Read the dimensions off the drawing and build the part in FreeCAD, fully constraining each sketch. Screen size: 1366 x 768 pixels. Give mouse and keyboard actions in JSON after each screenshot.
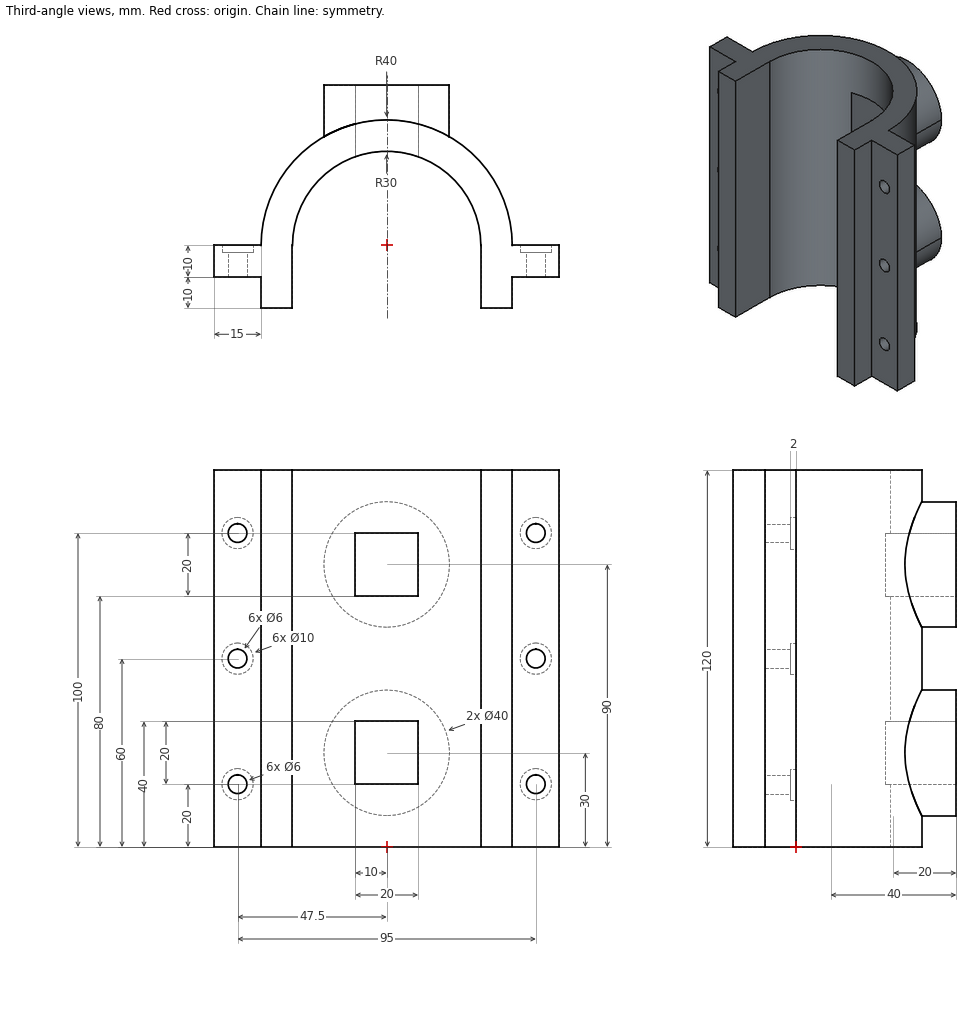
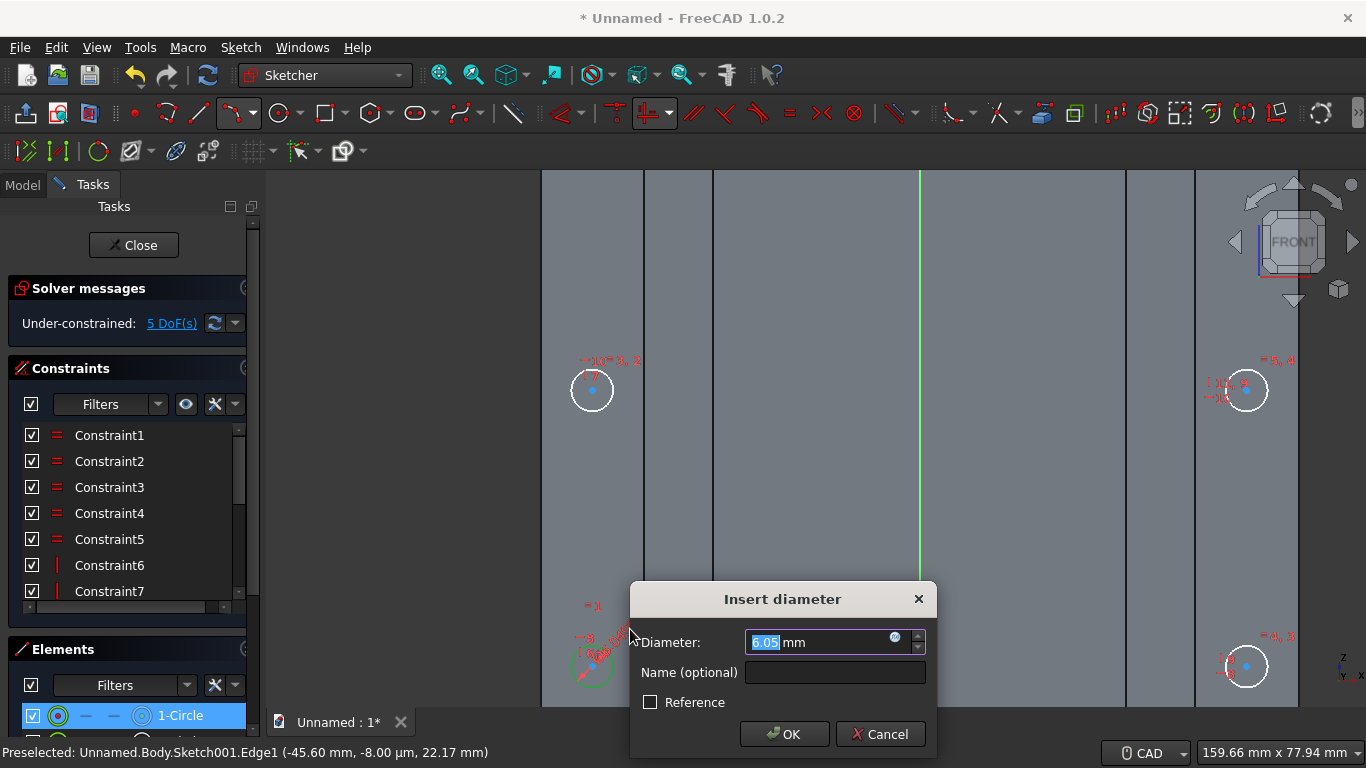
{"action": "type", "text": "6"}
{"action": "key", "text": "Return"}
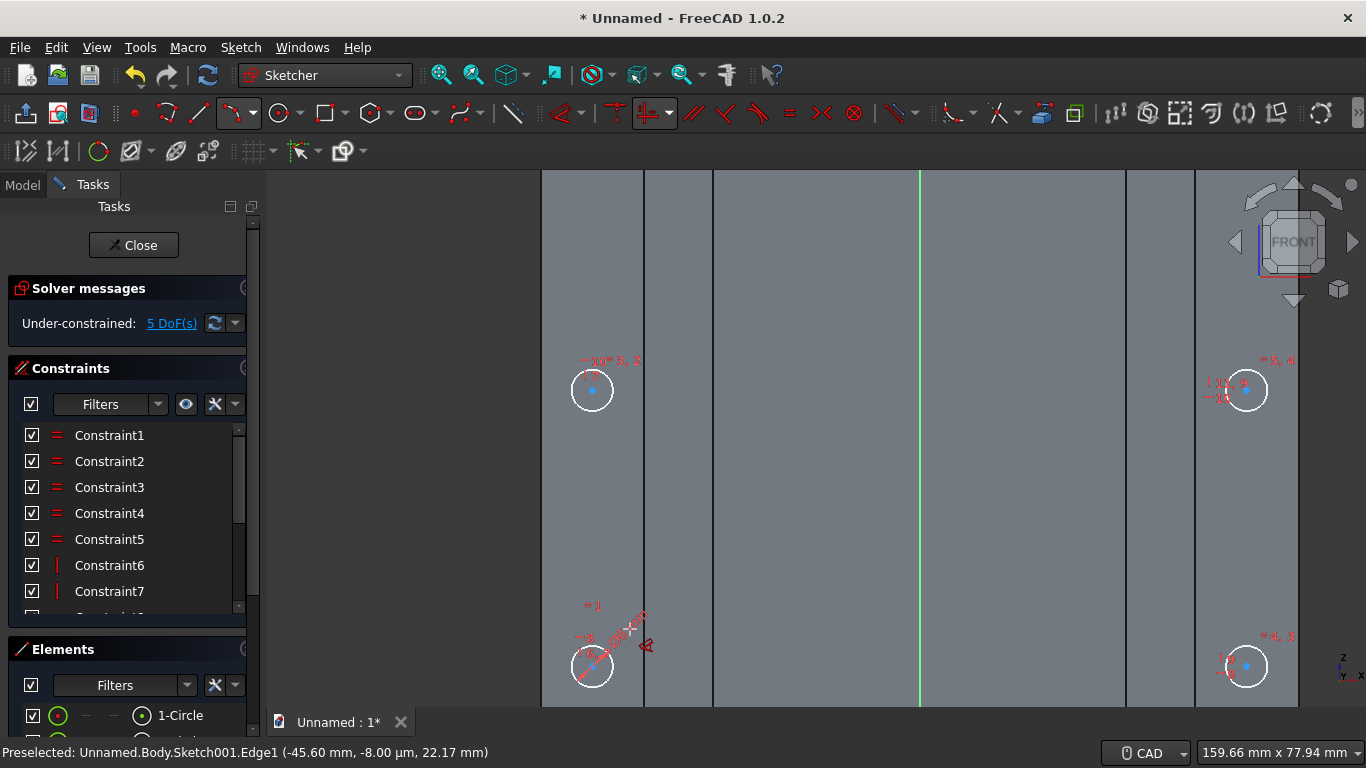
{"action": "left_click", "coordinate": [592, 667]}
{"action": "left_click", "coordinate": [558, 673]}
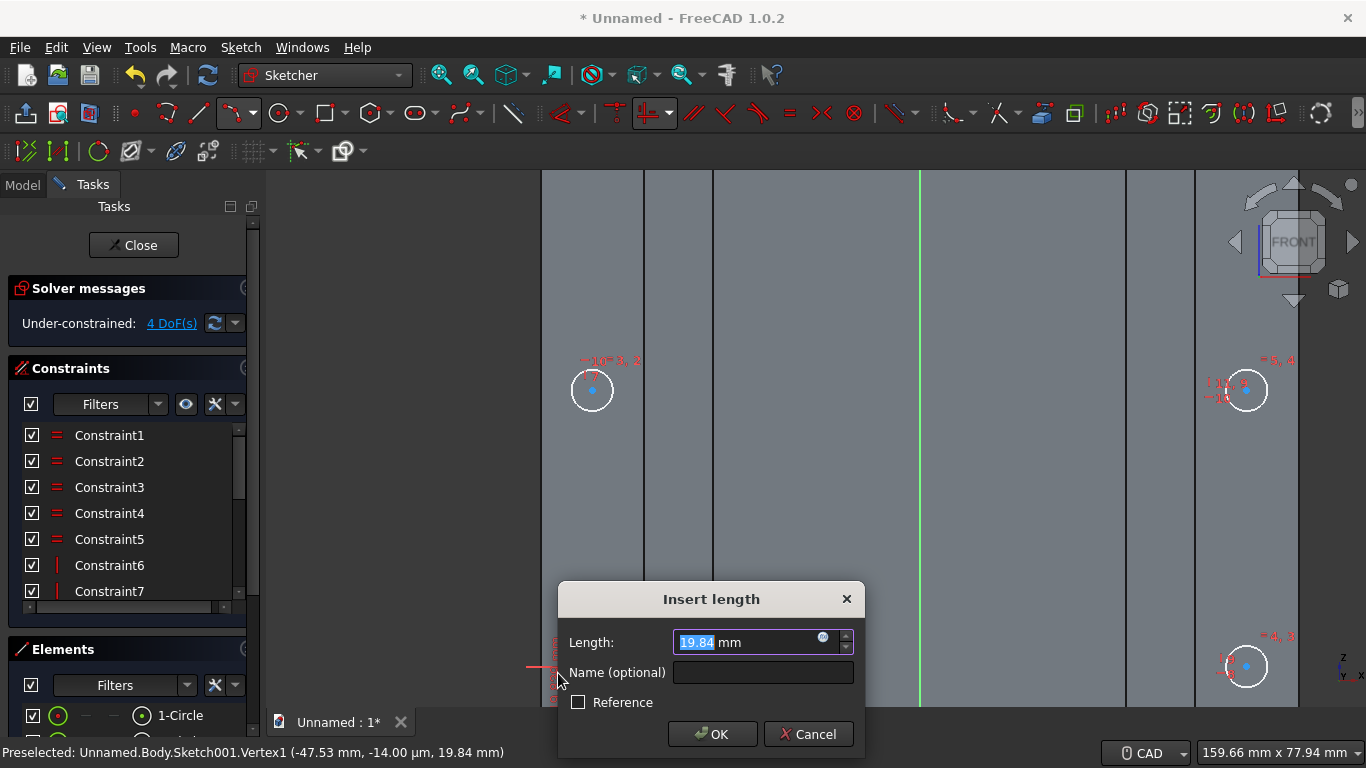
{"action": "type", "text": "20"}
{"action": "key", "text": "Return"}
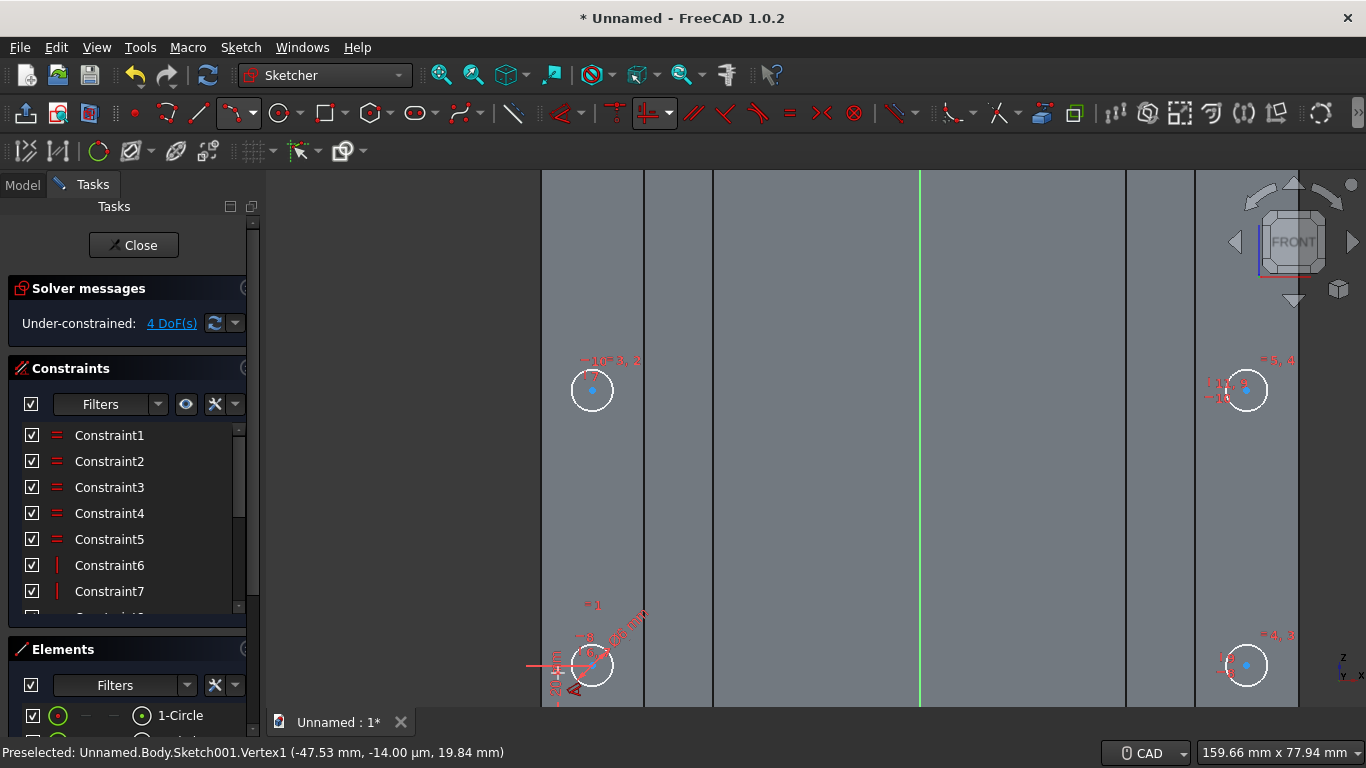
{"action": "left_click", "coordinate": [592, 390]}
{"action": "left_click", "coordinate": [558, 535]}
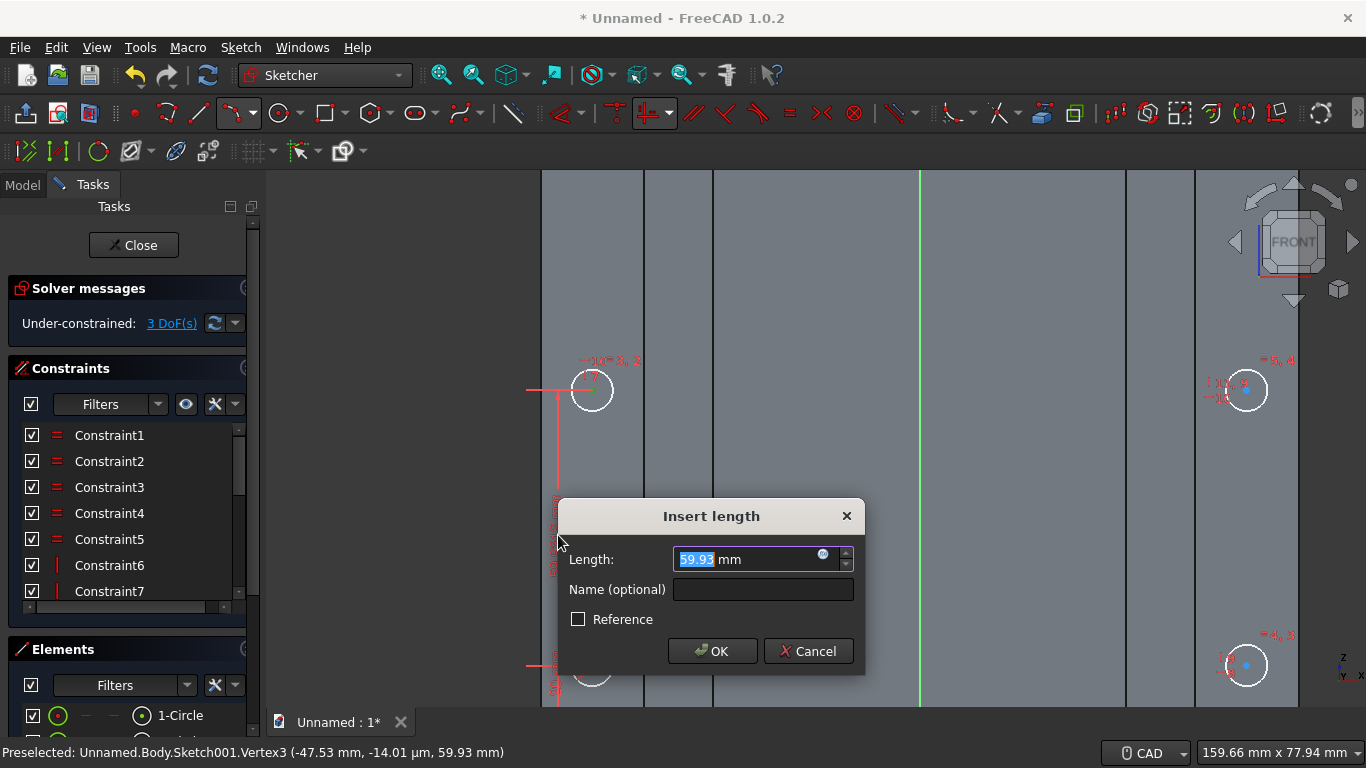
{"action": "type", "text": "60"}
{"action": "key", "text": "Return"}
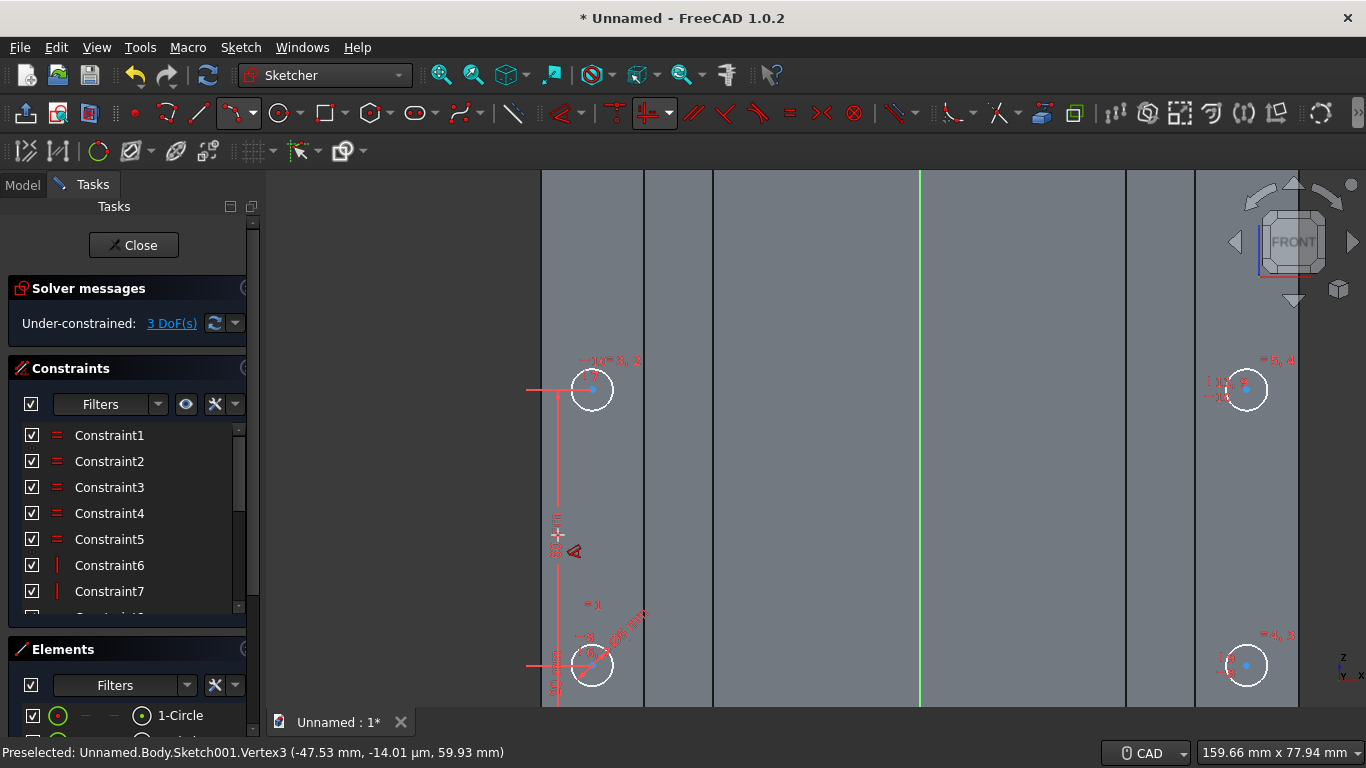
{"action": "scroll", "coordinate": [607, 430], "scroll_direction": "down", "scroll_amount": 4}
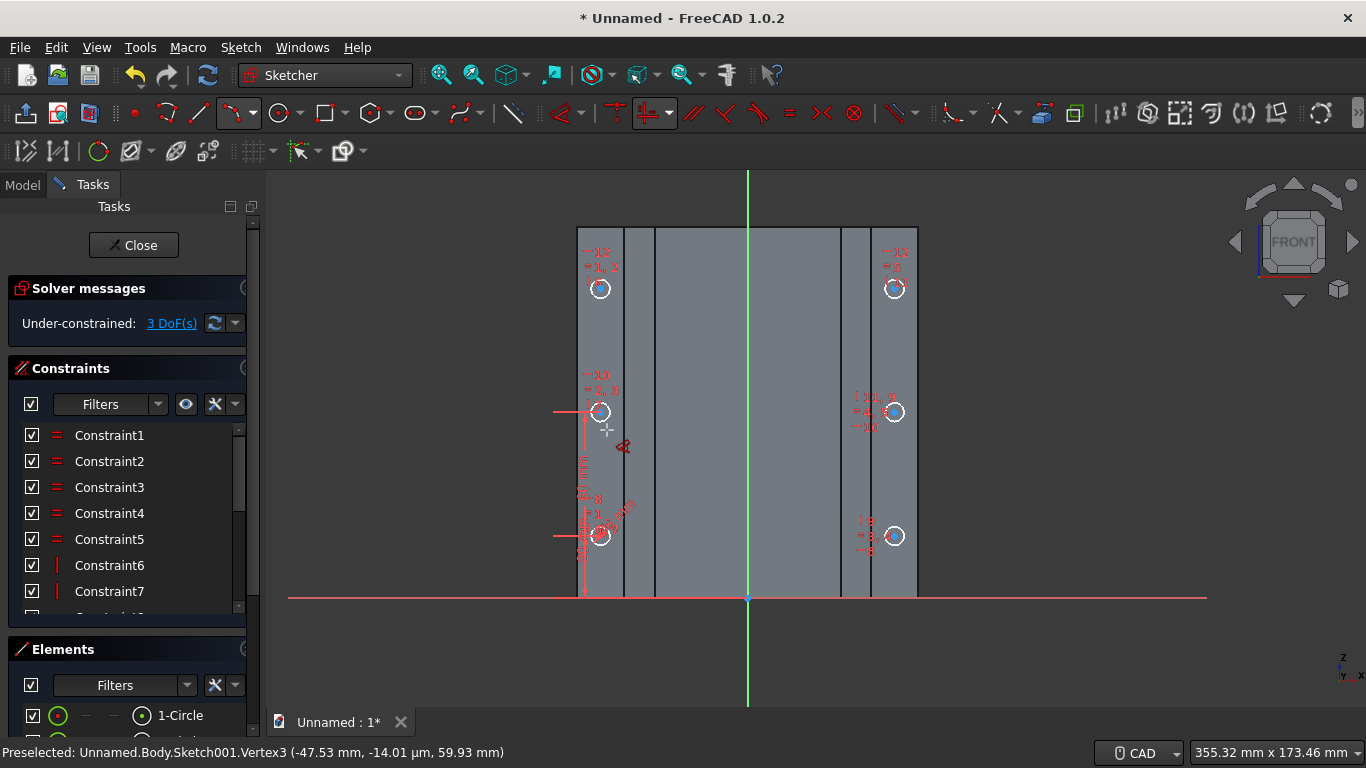
{"action": "left_click", "coordinate": [601, 289]}
{"action": "left_click", "coordinate": [567, 443]}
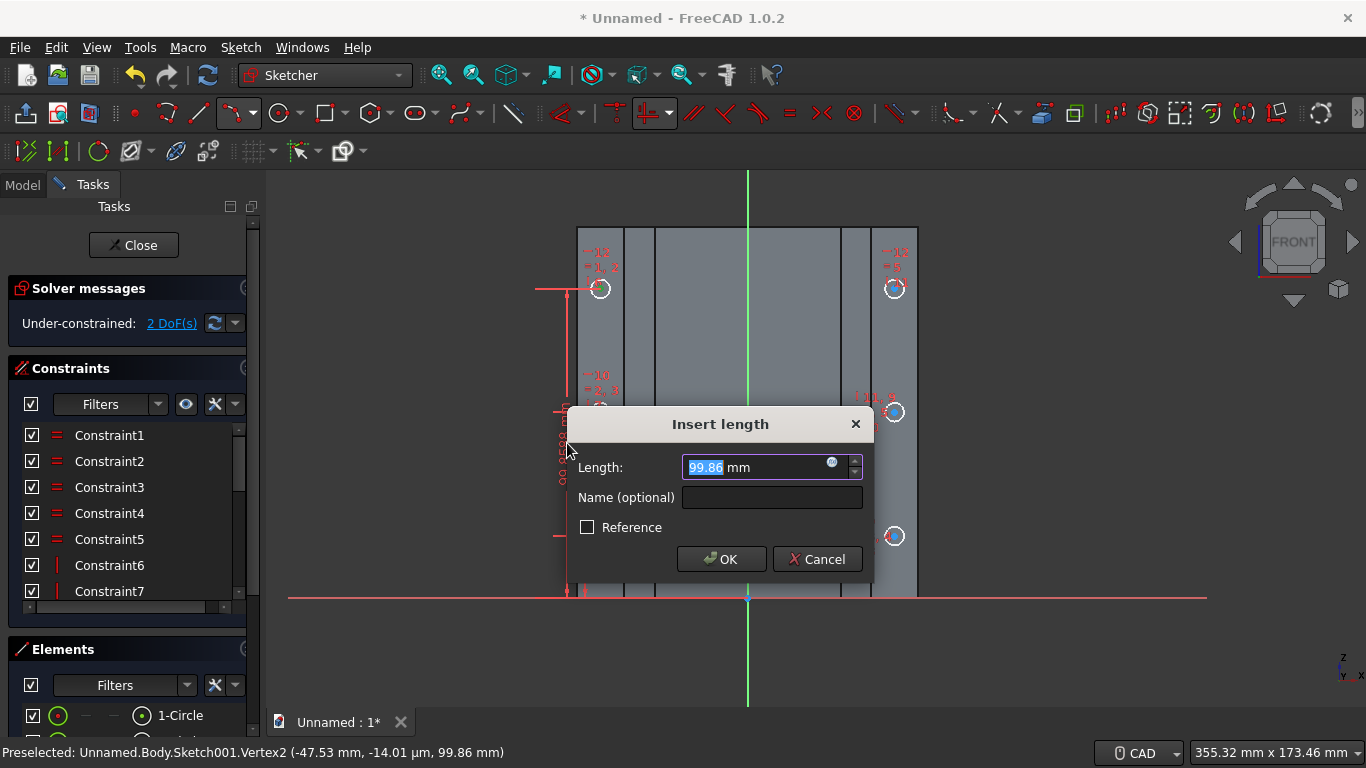
{"action": "type", "text": "100"}
{"action": "key", "text": "Return"}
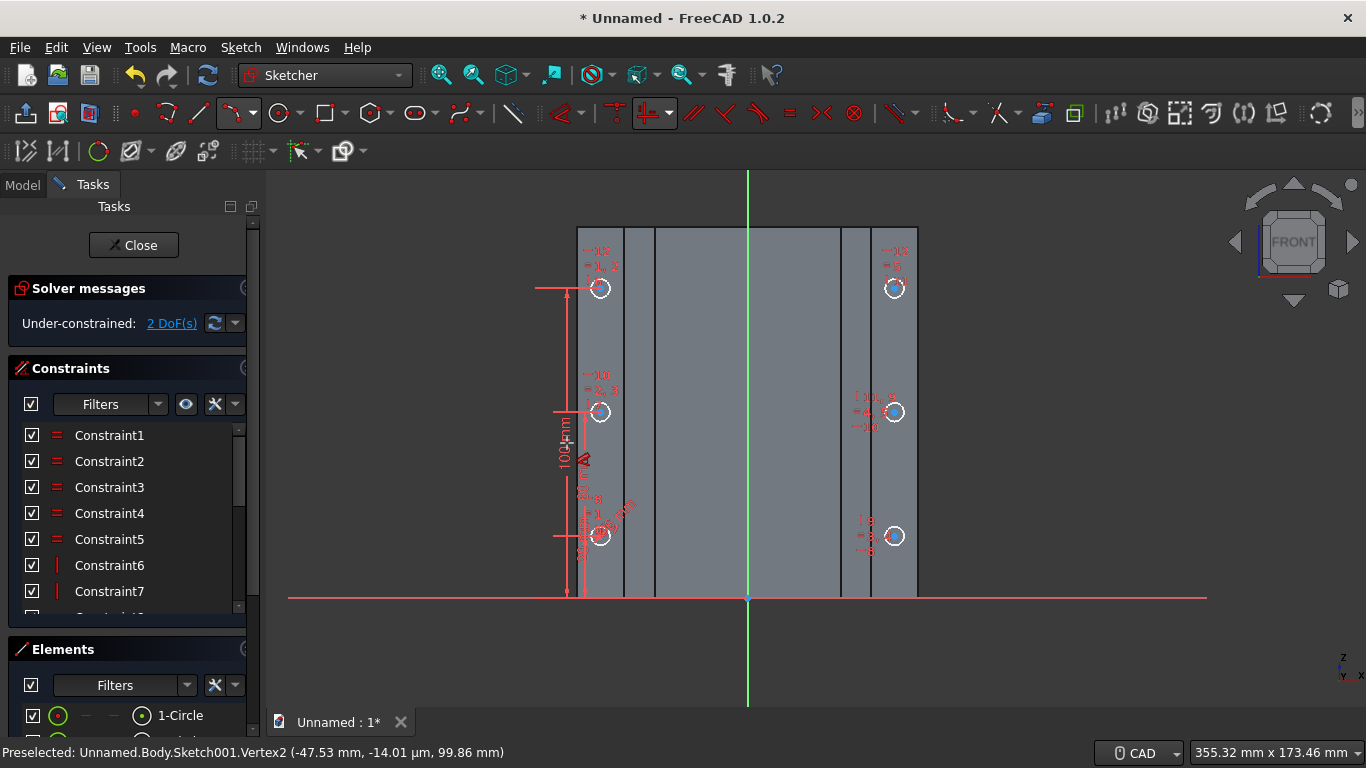
{"action": "left_click", "coordinate": [601, 536]}